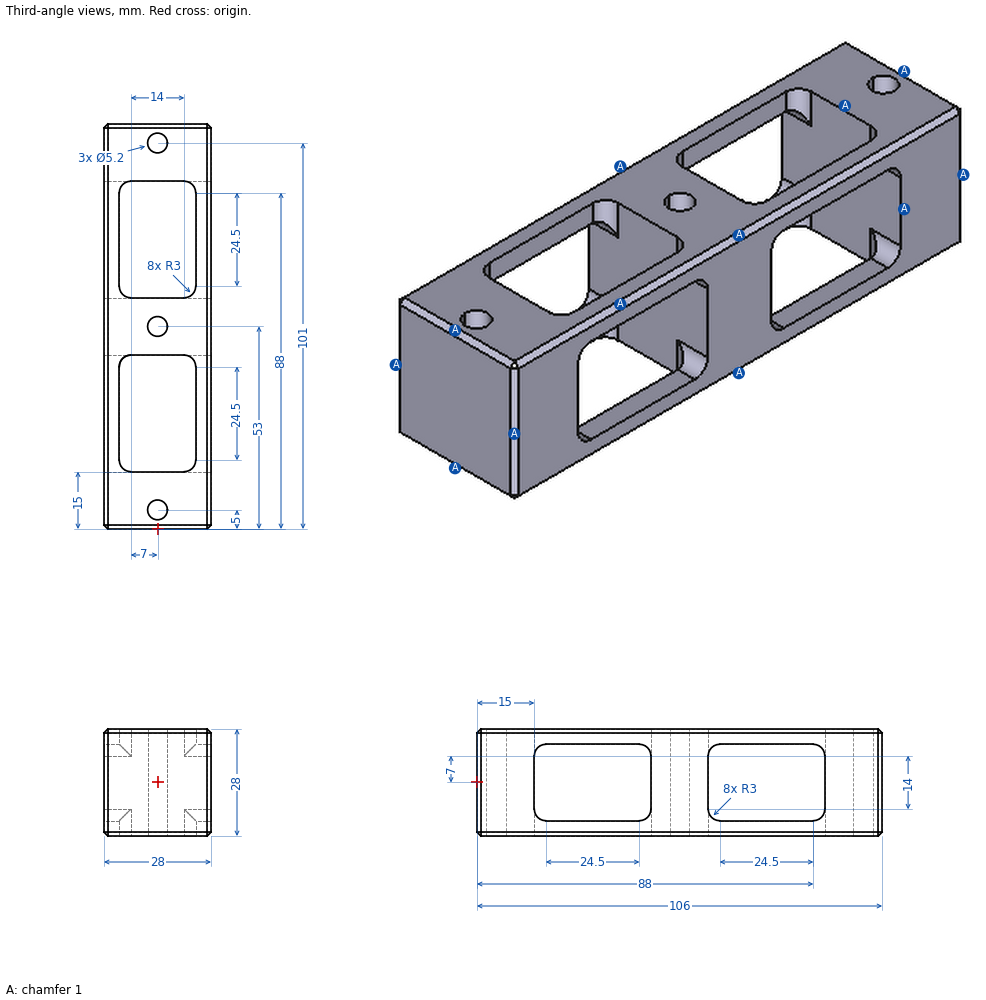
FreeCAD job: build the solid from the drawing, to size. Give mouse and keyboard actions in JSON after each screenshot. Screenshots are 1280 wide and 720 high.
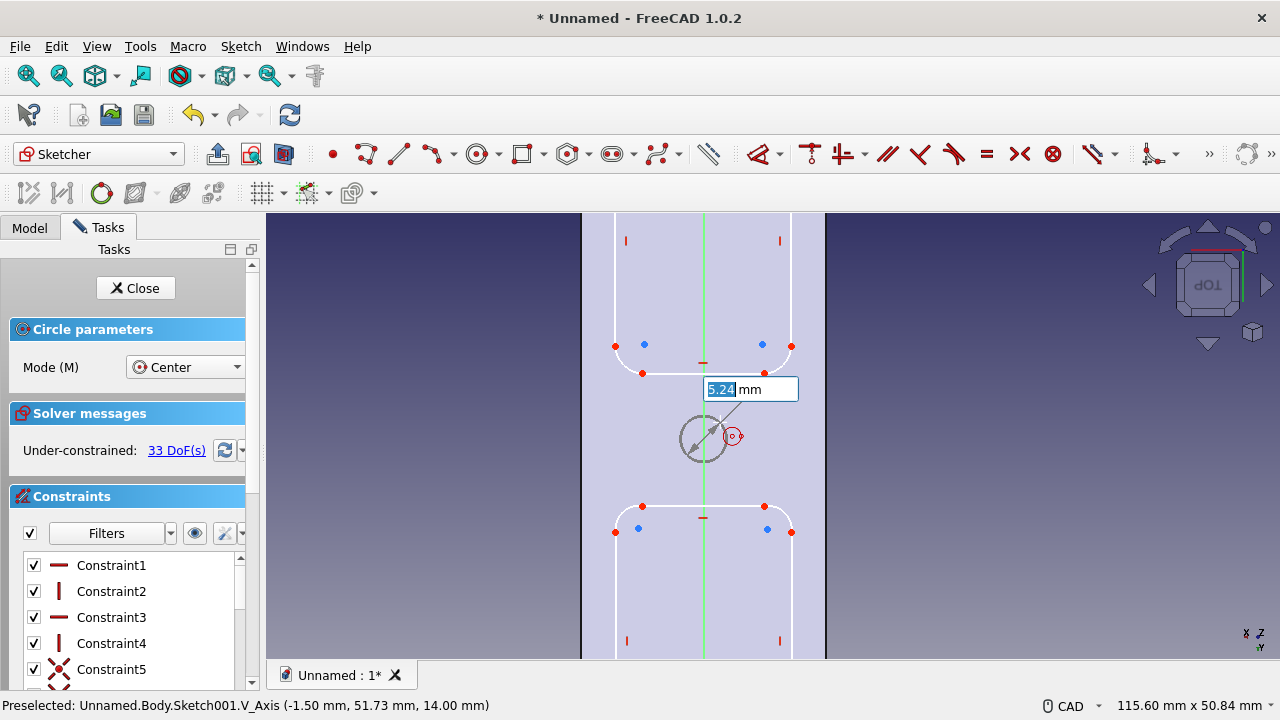
{"action": "type", "text": "5.2"}
{"action": "key", "text": "Return"}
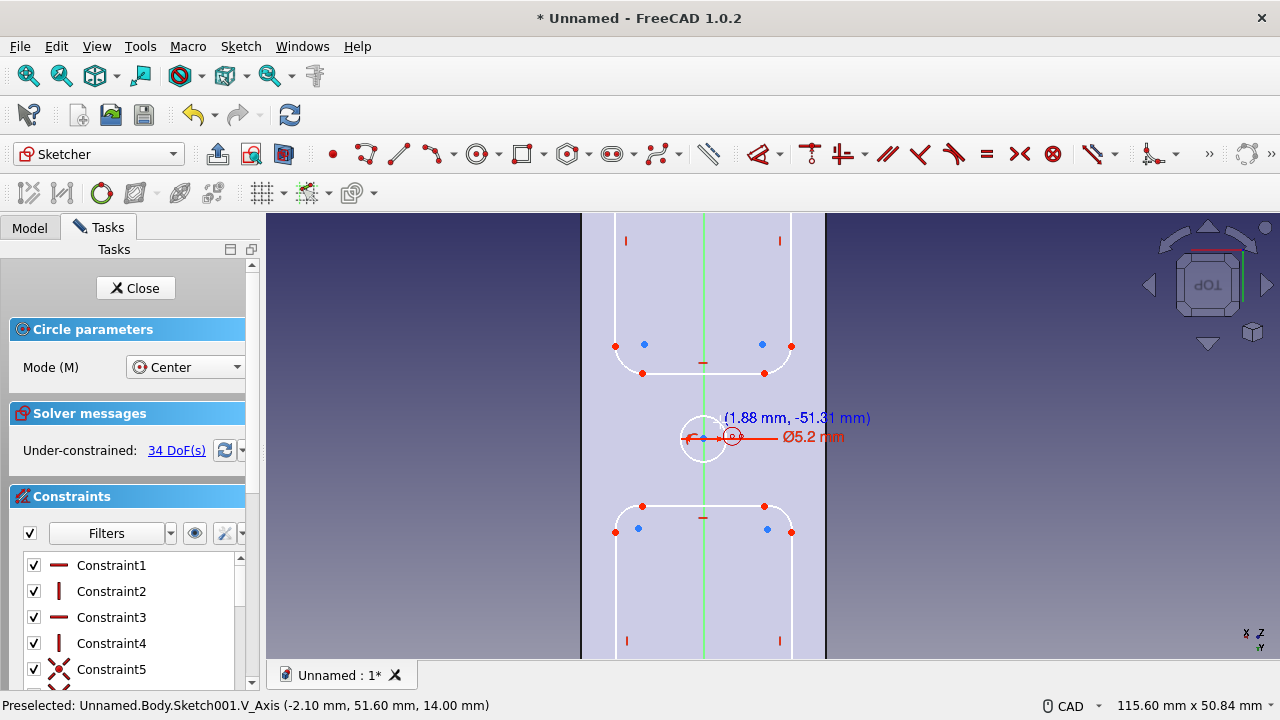
{"action": "scroll", "coordinate": [705, 440], "scroll_direction": "down", "scroll_amount": 6}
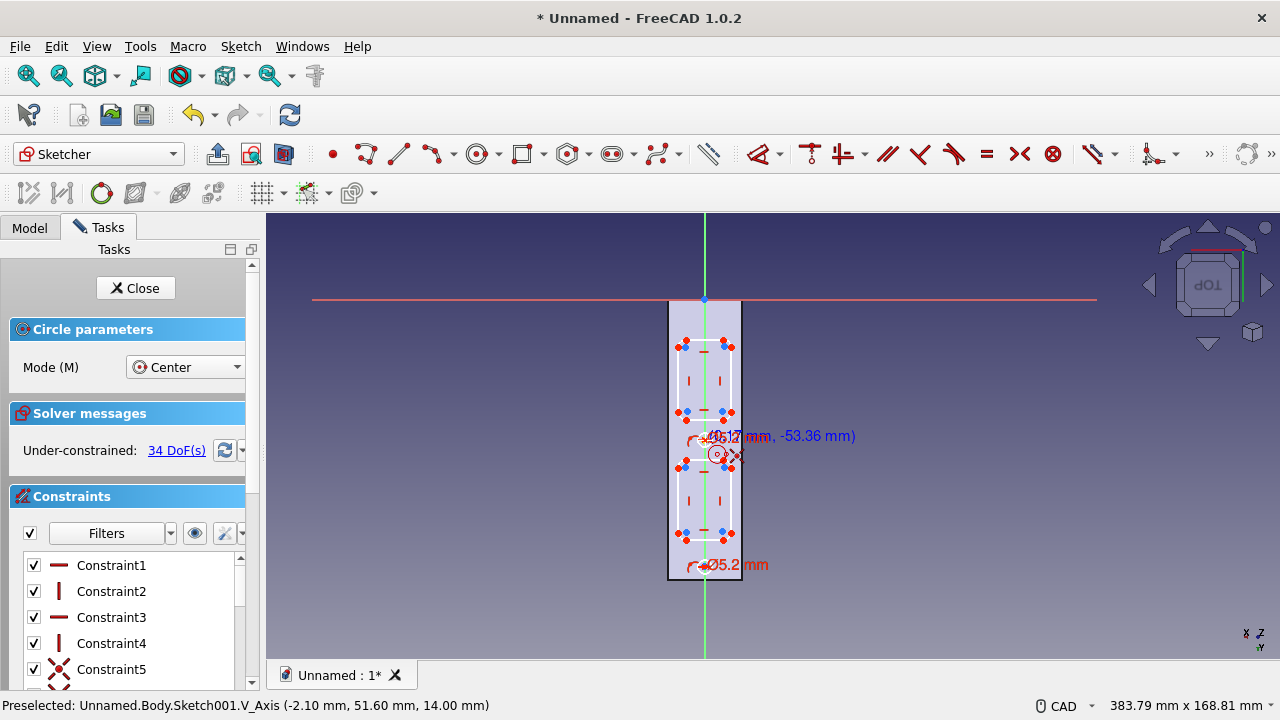
{"action": "scroll", "coordinate": [705, 313], "scroll_direction": "up", "scroll_amount": 6}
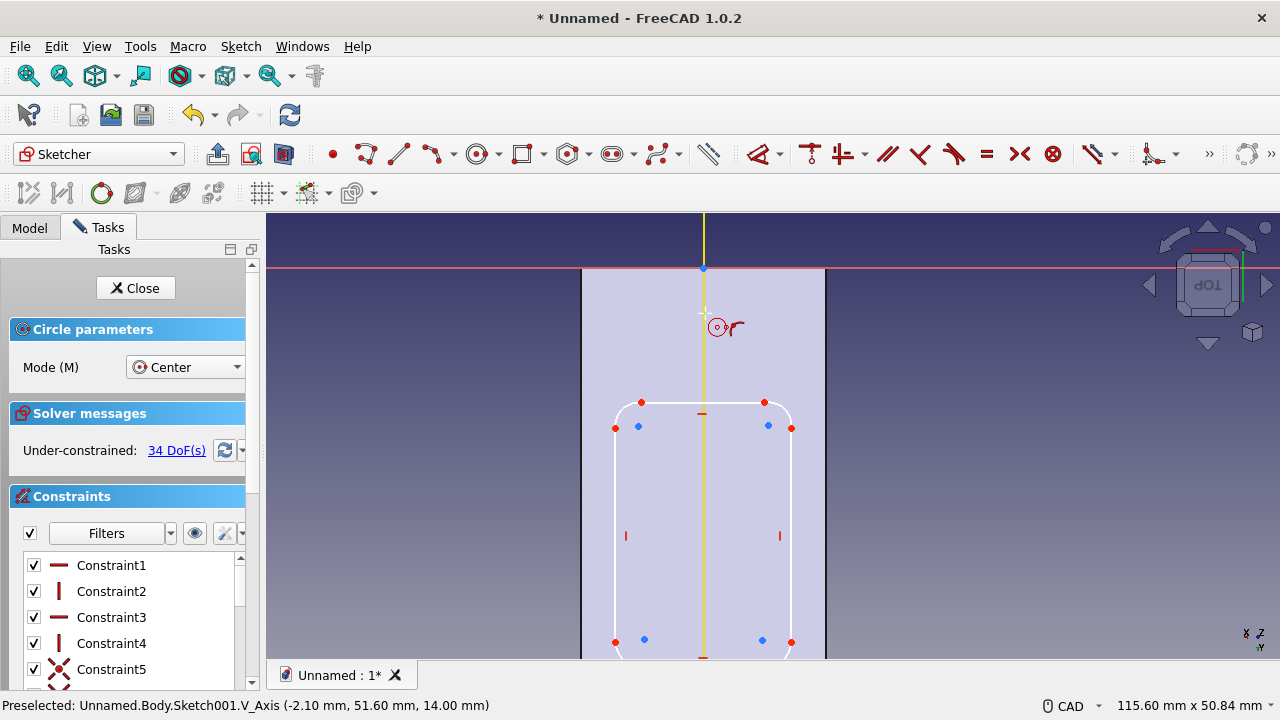
{"action": "left_click", "coordinate": [704, 312]}
{"action": "mouse_move", "coordinate": [720, 296]}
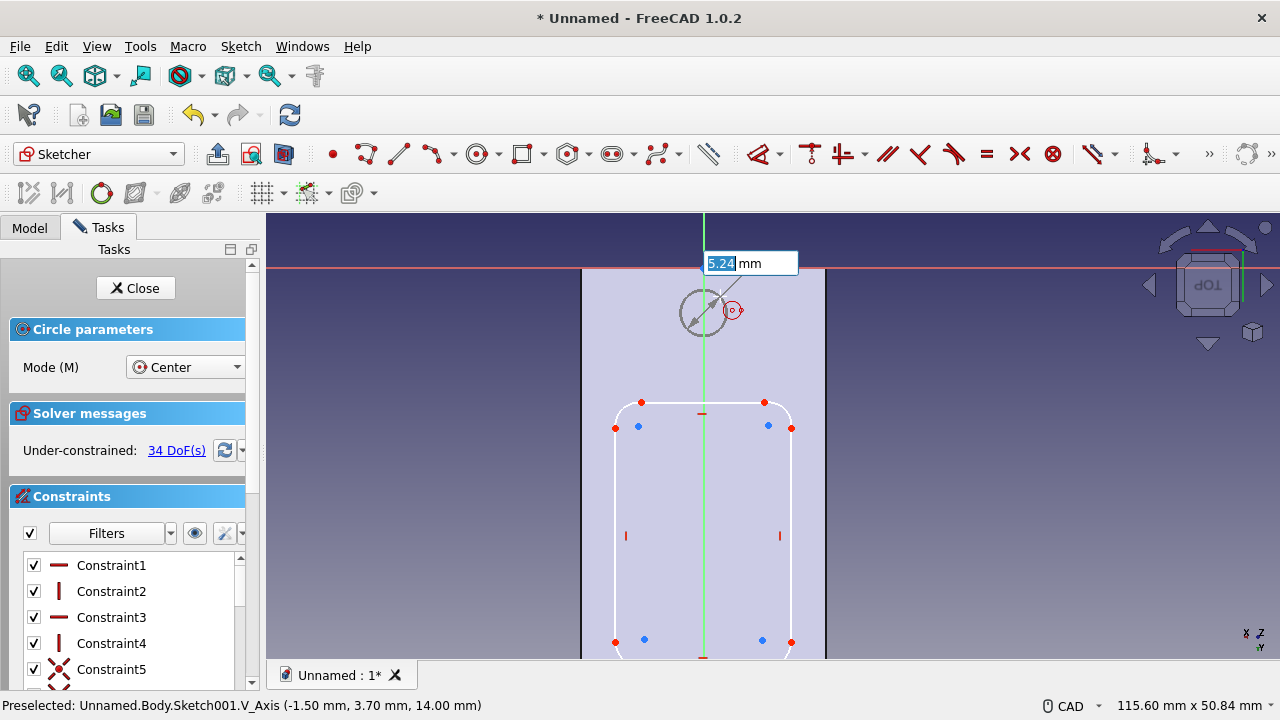
{"action": "type", "text": "5.2"}
{"action": "key", "text": "Return"}
{"action": "key", "text": "Escape"}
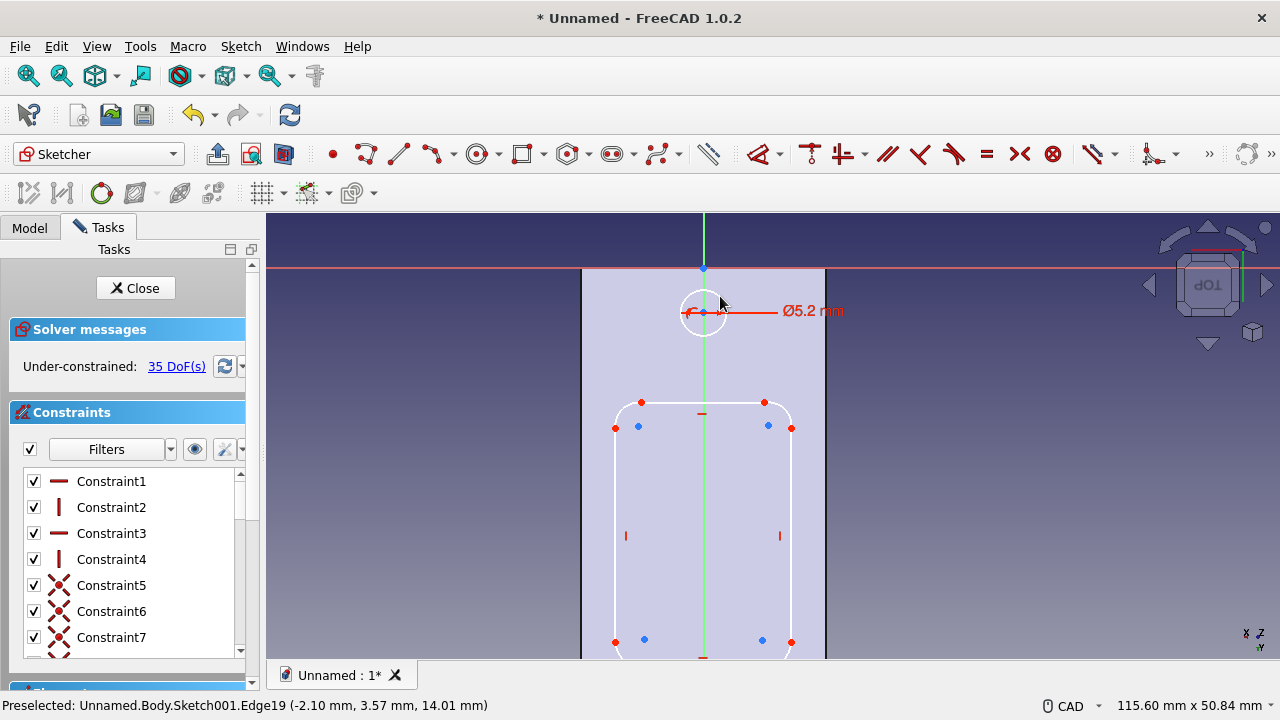
{"action": "scroll", "coordinate": [705, 312], "scroll_direction": "down", "scroll_amount": 6}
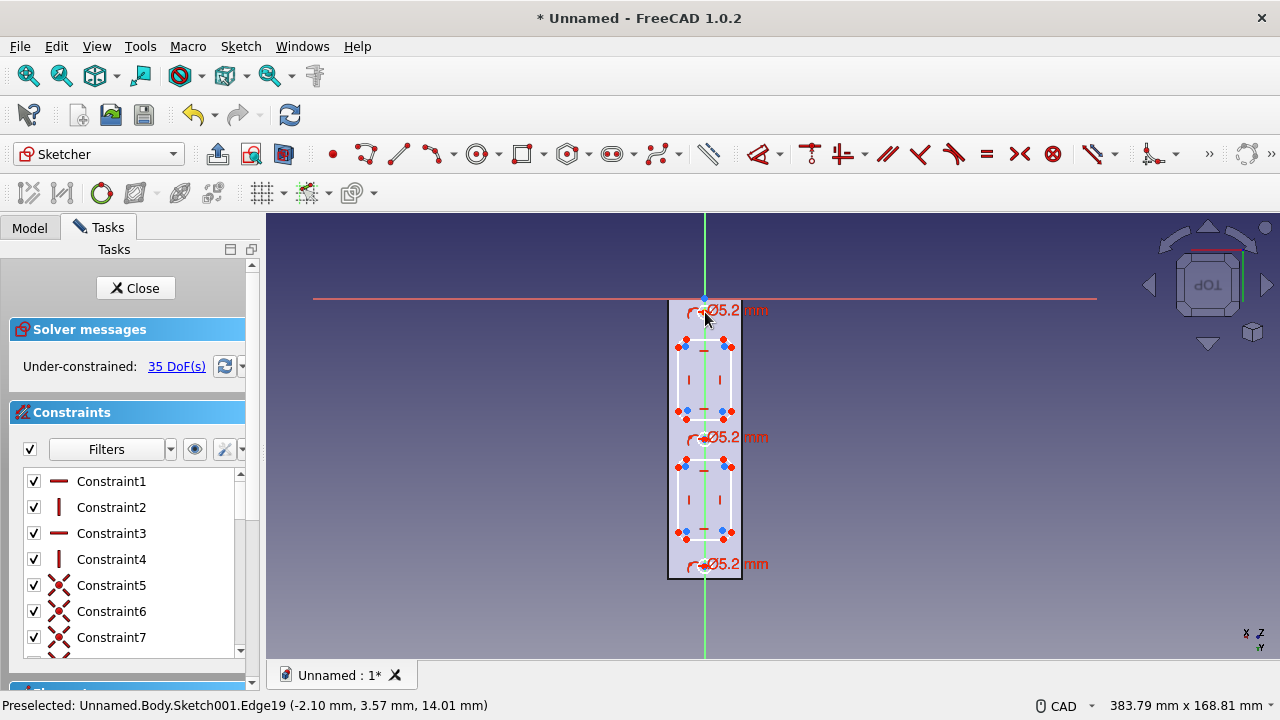
{"action": "scroll", "coordinate": [712, 460], "scroll_direction": "up", "scroll_amount": 4}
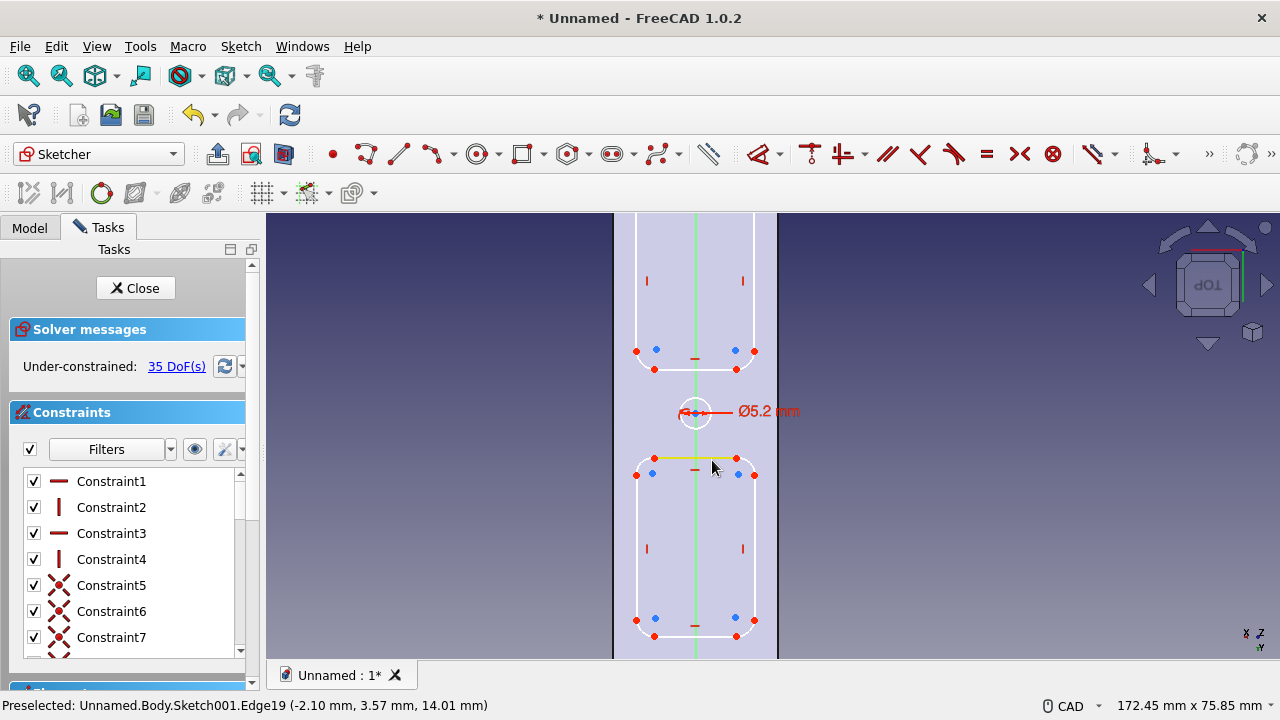
{"action": "left_click", "coordinate": [712, 458]}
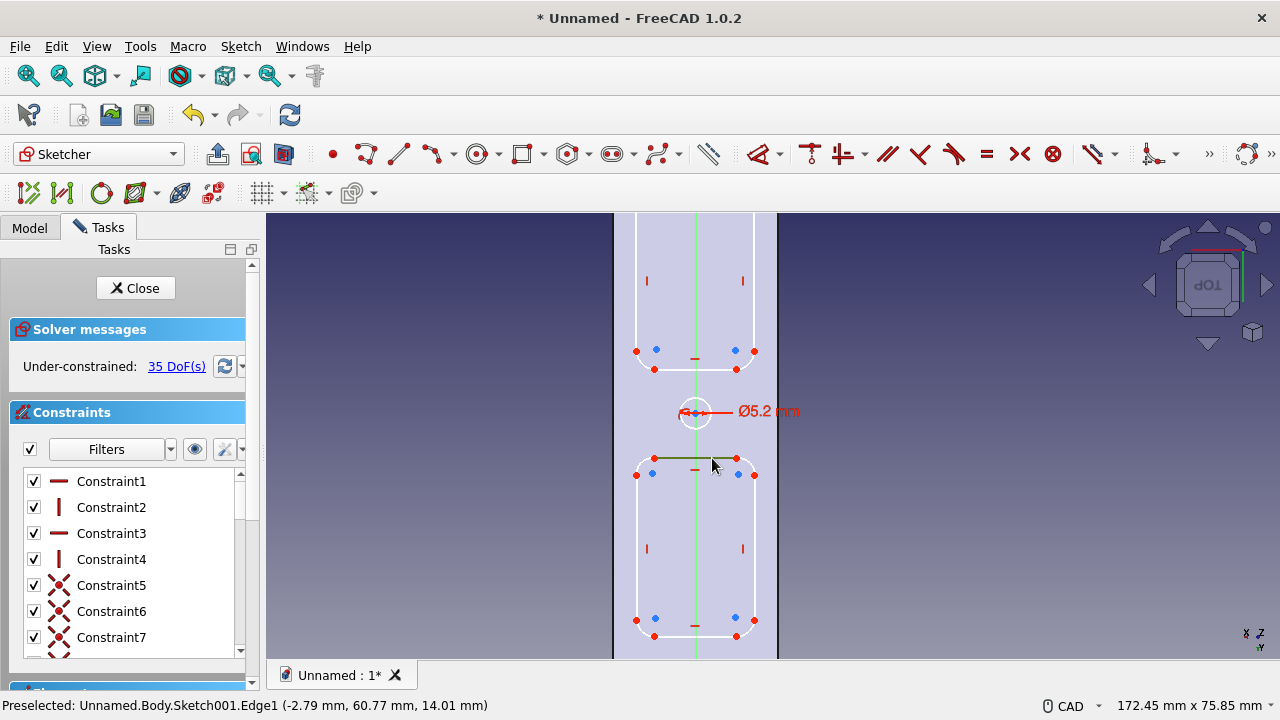
{"action": "left_click", "coordinate": [641, 463]}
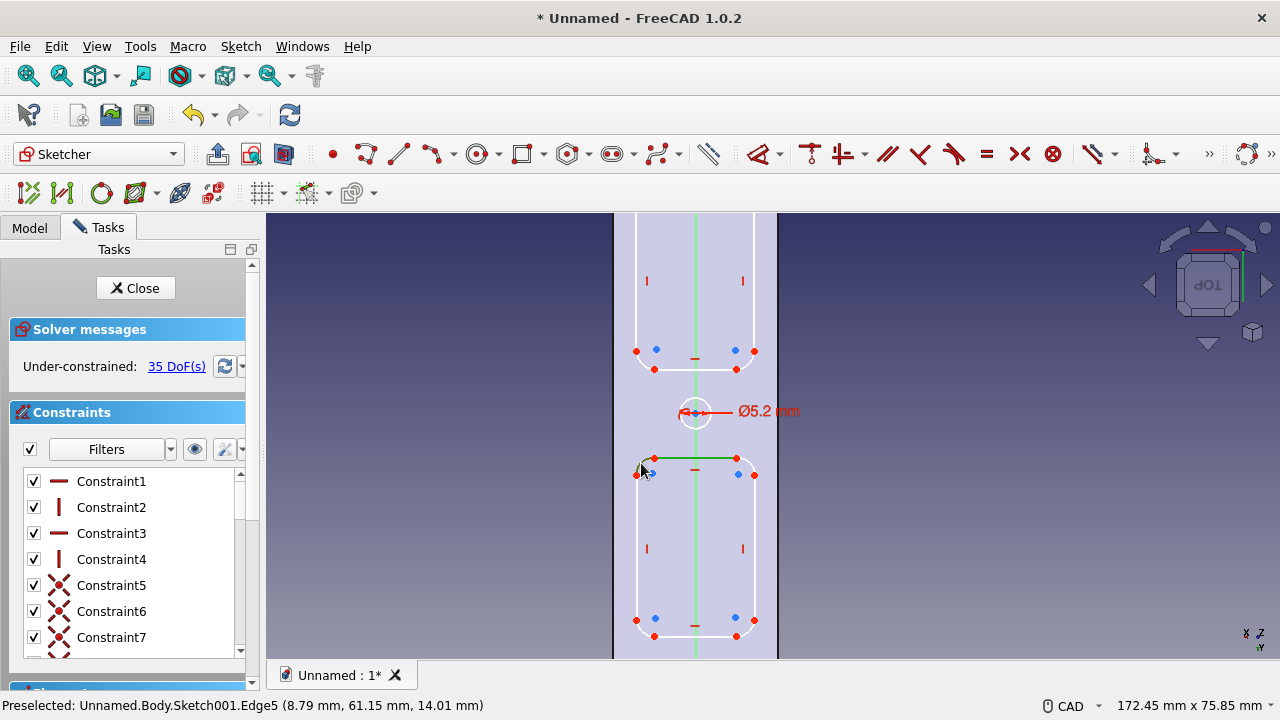
{"action": "left_click", "coordinate": [954, 154]}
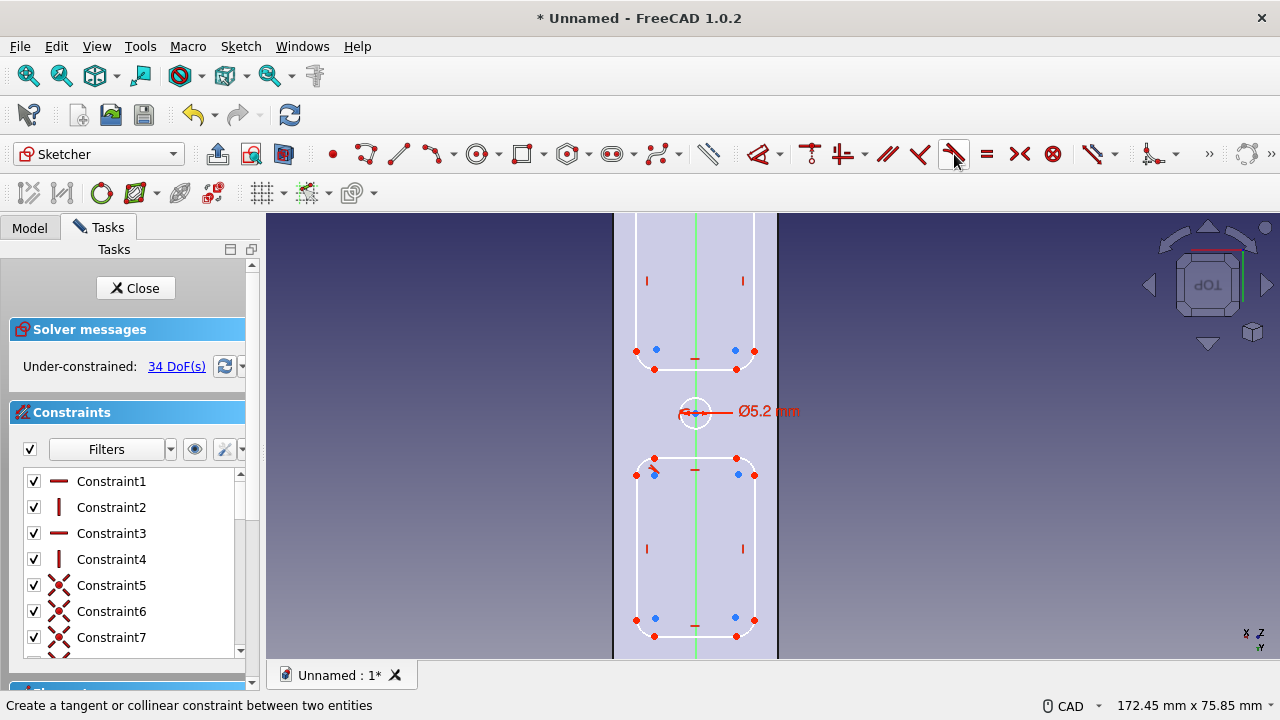
{"action": "left_click", "coordinate": [712, 458]}